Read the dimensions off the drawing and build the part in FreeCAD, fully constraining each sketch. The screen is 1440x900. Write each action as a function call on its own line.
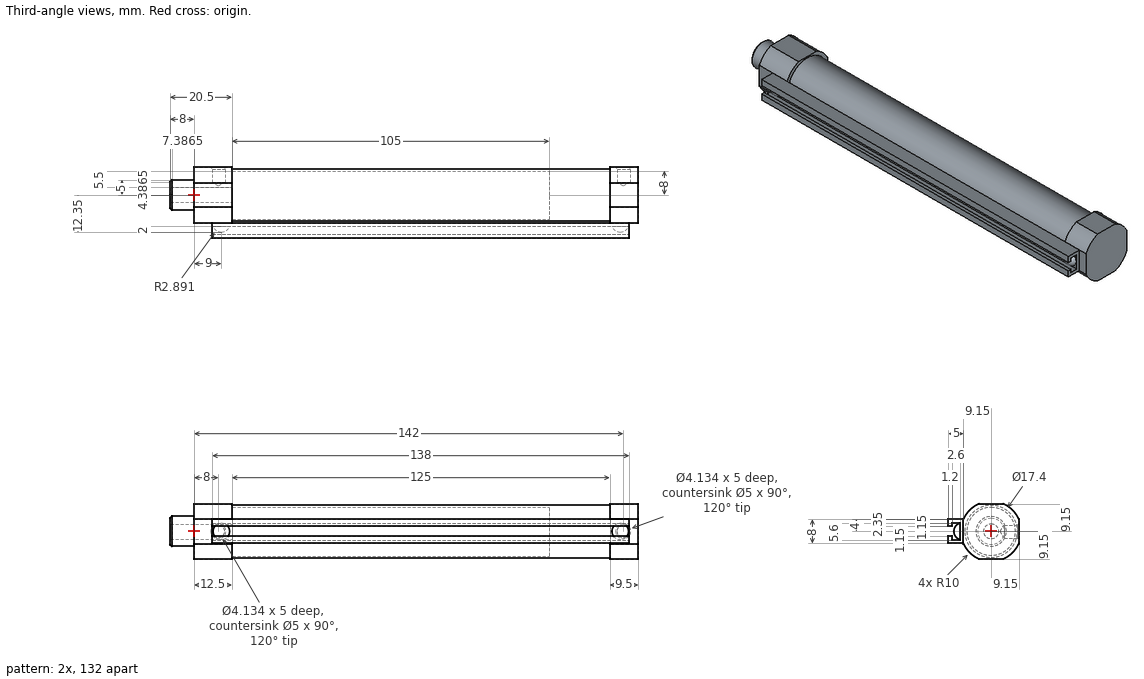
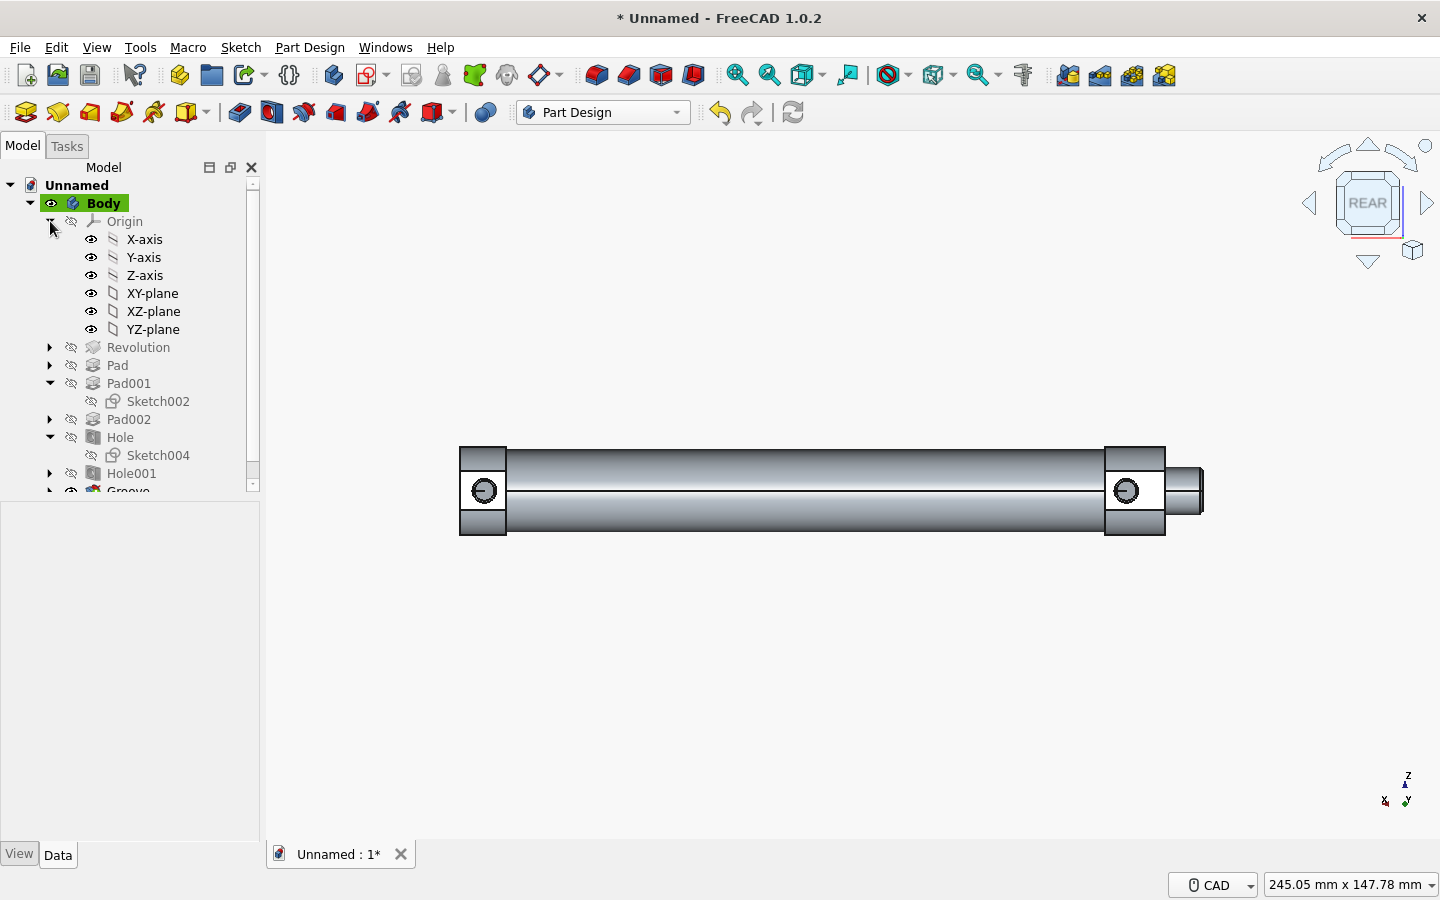
click(136, 329)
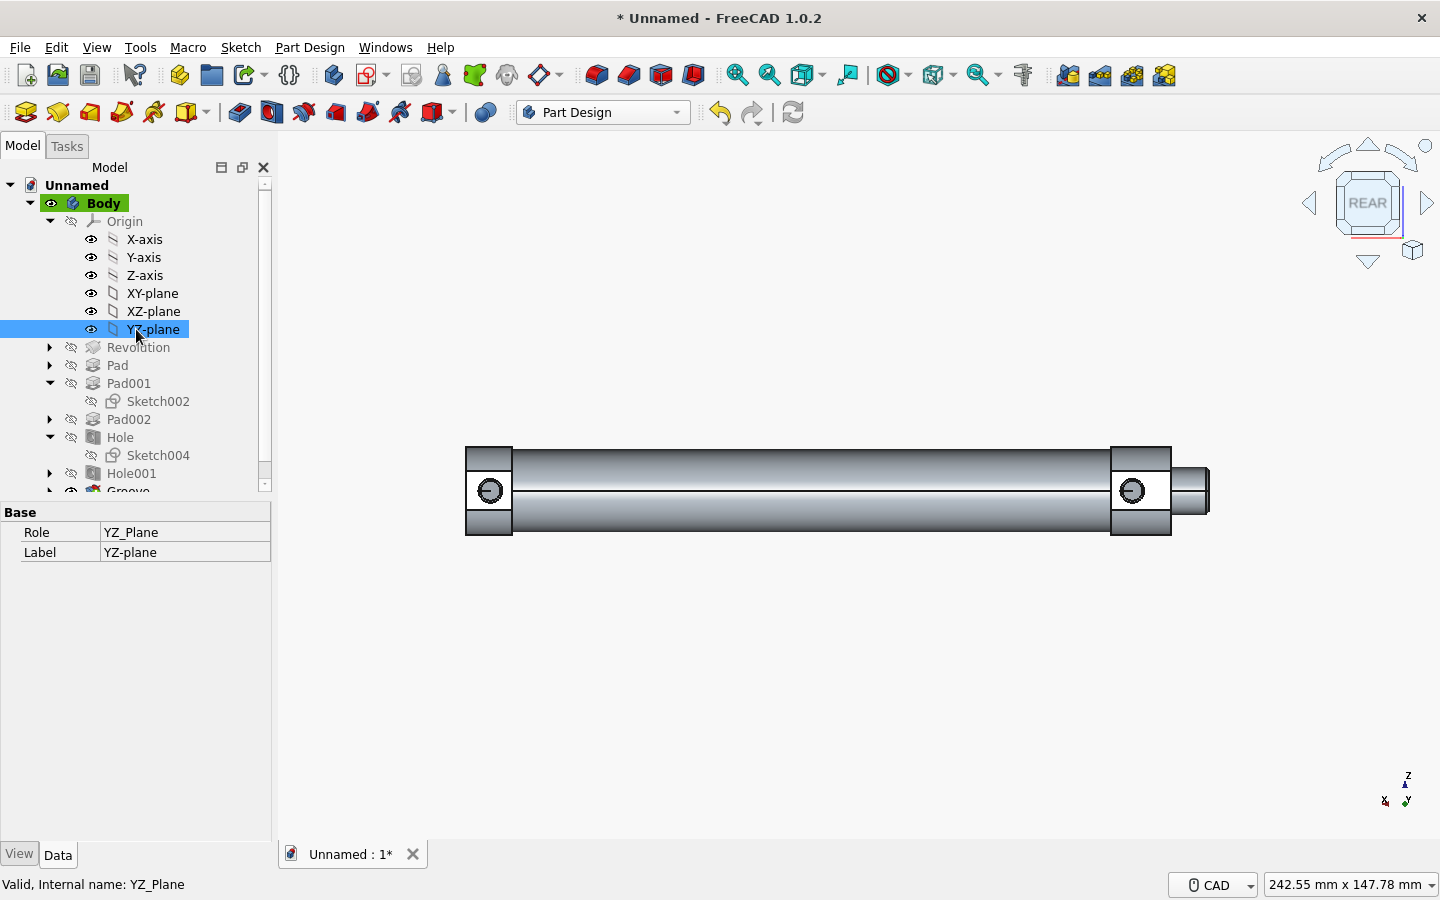
click(540, 76)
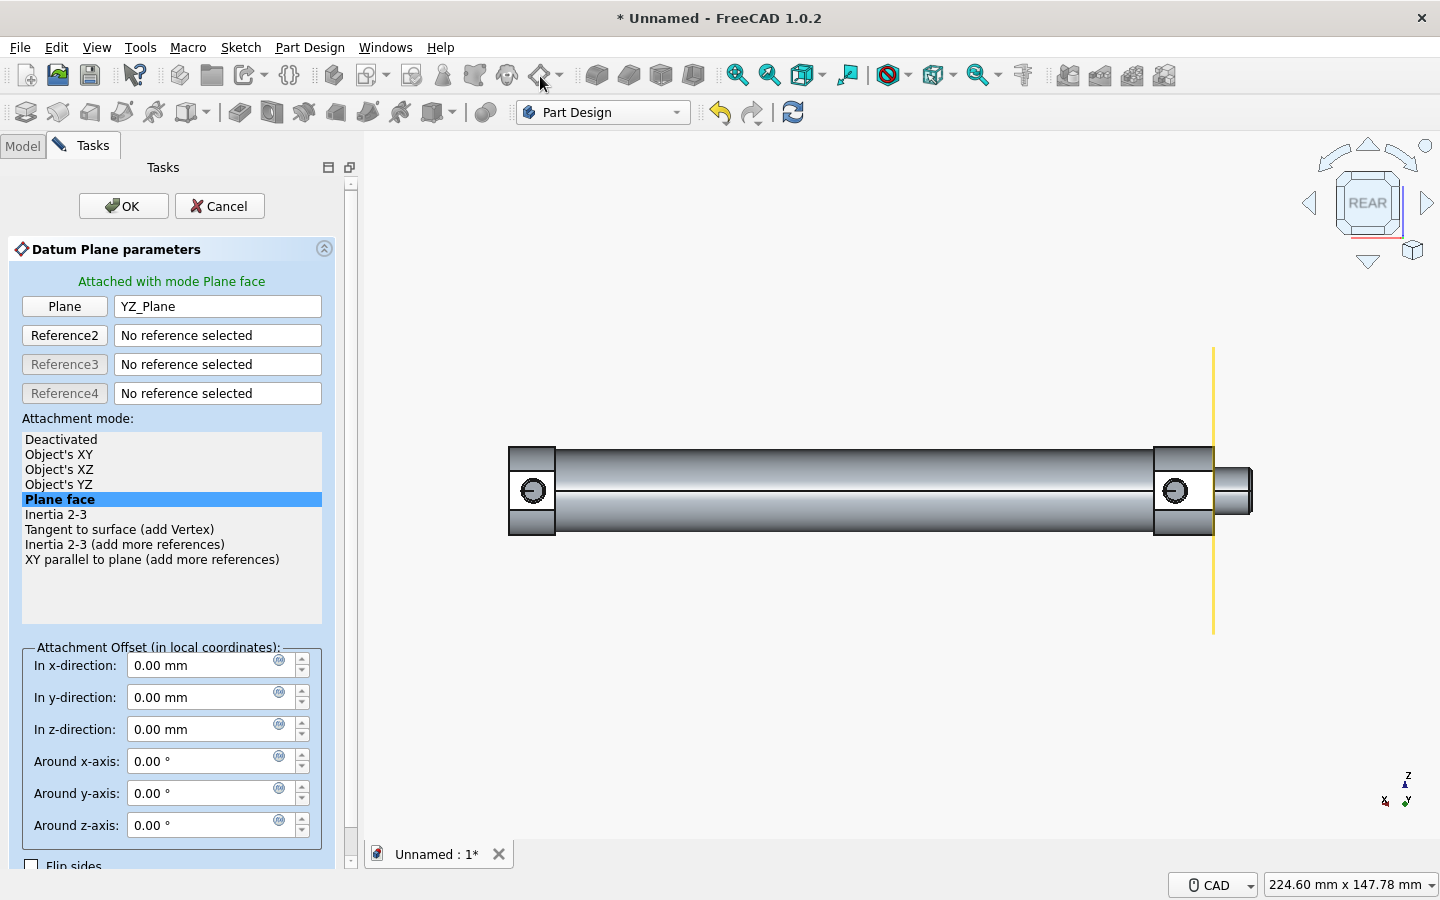
triple_click(210, 729)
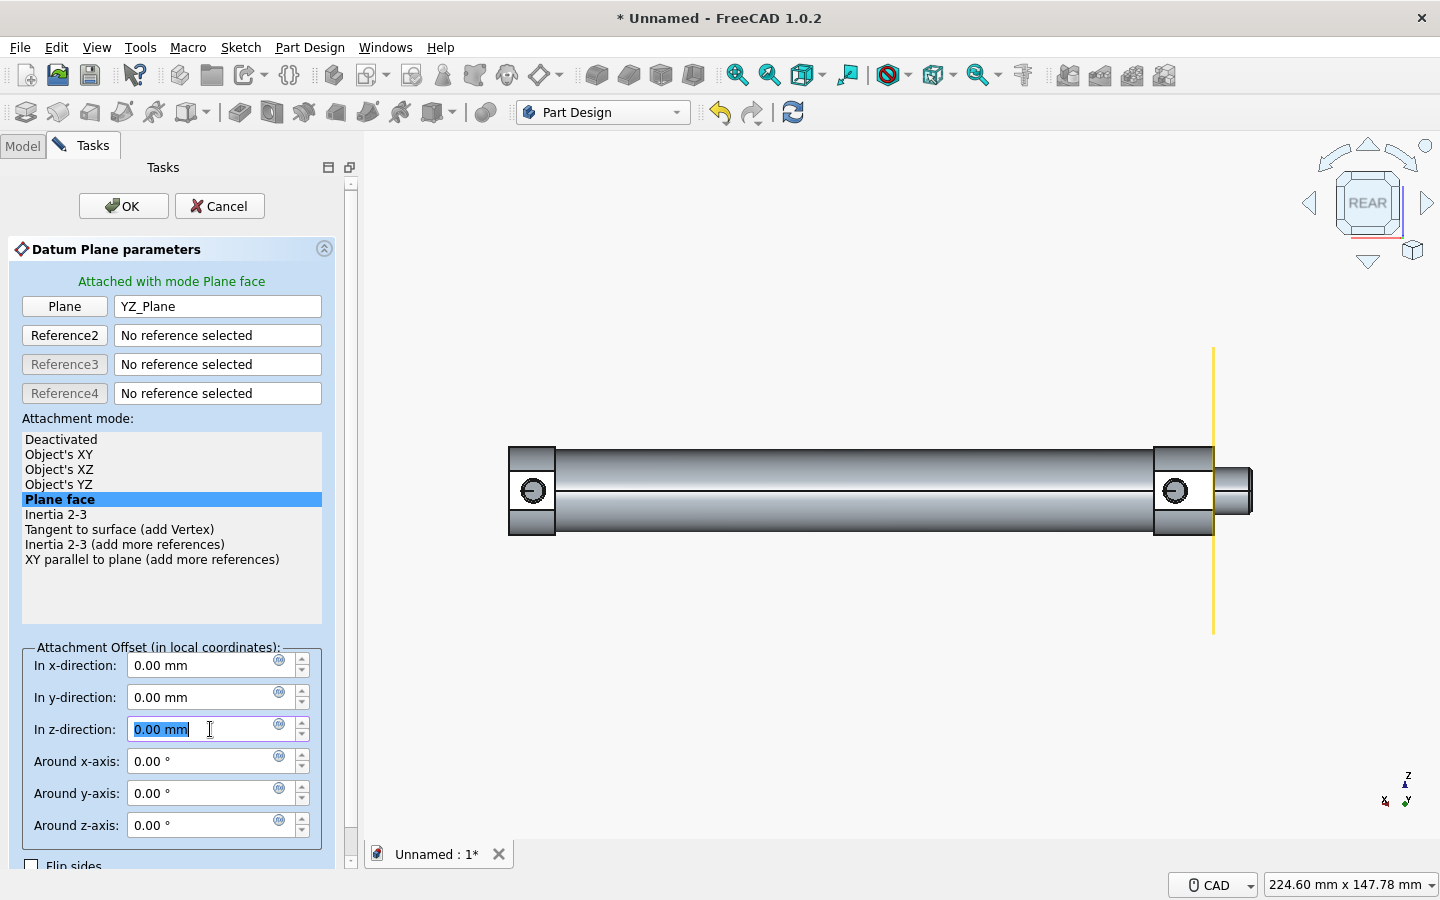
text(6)
key(Tab)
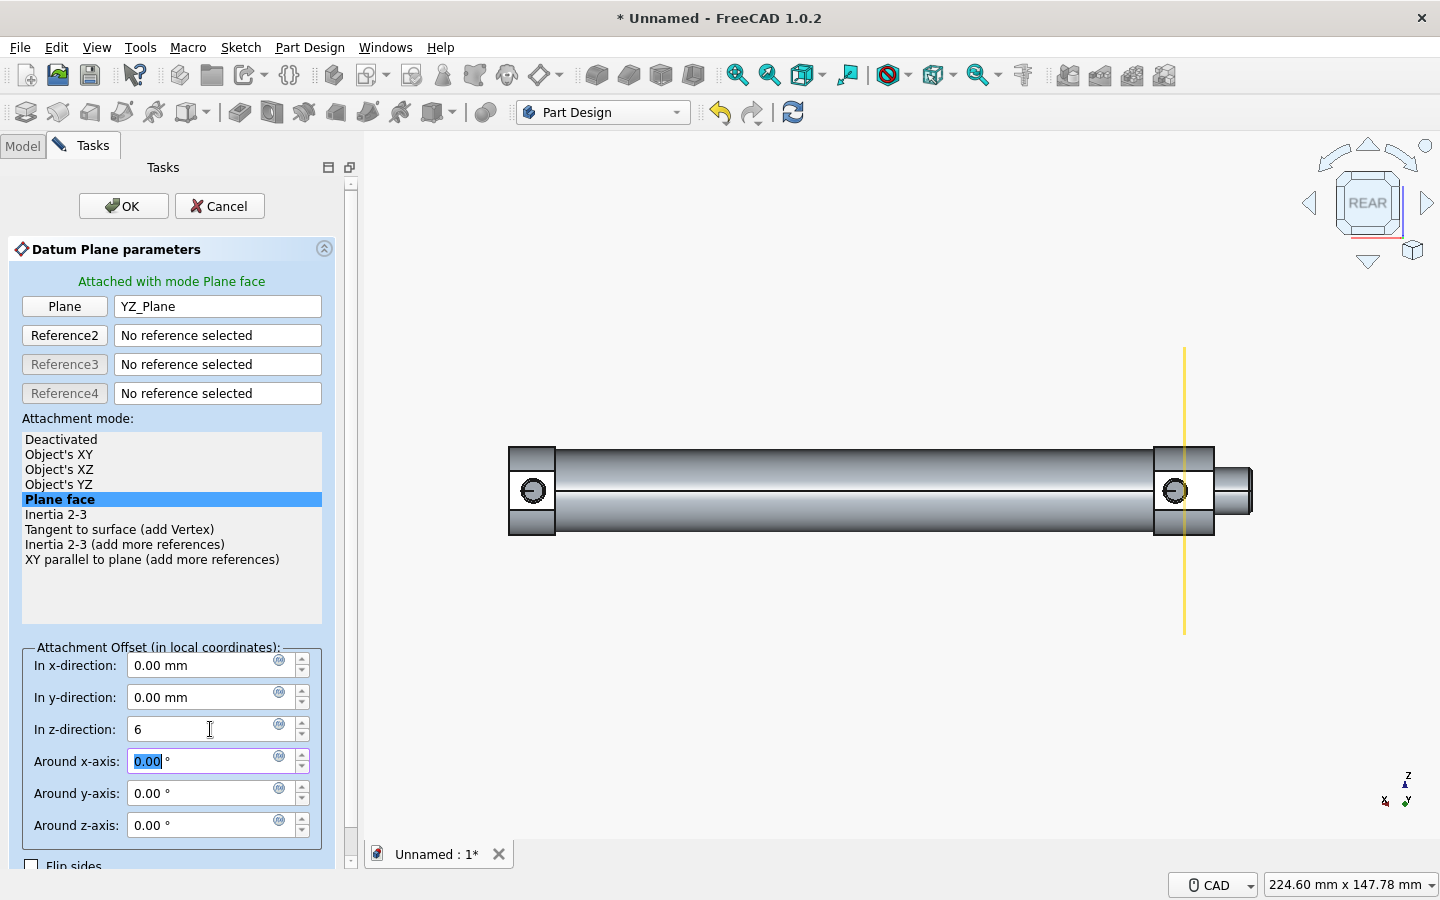
click(124, 206)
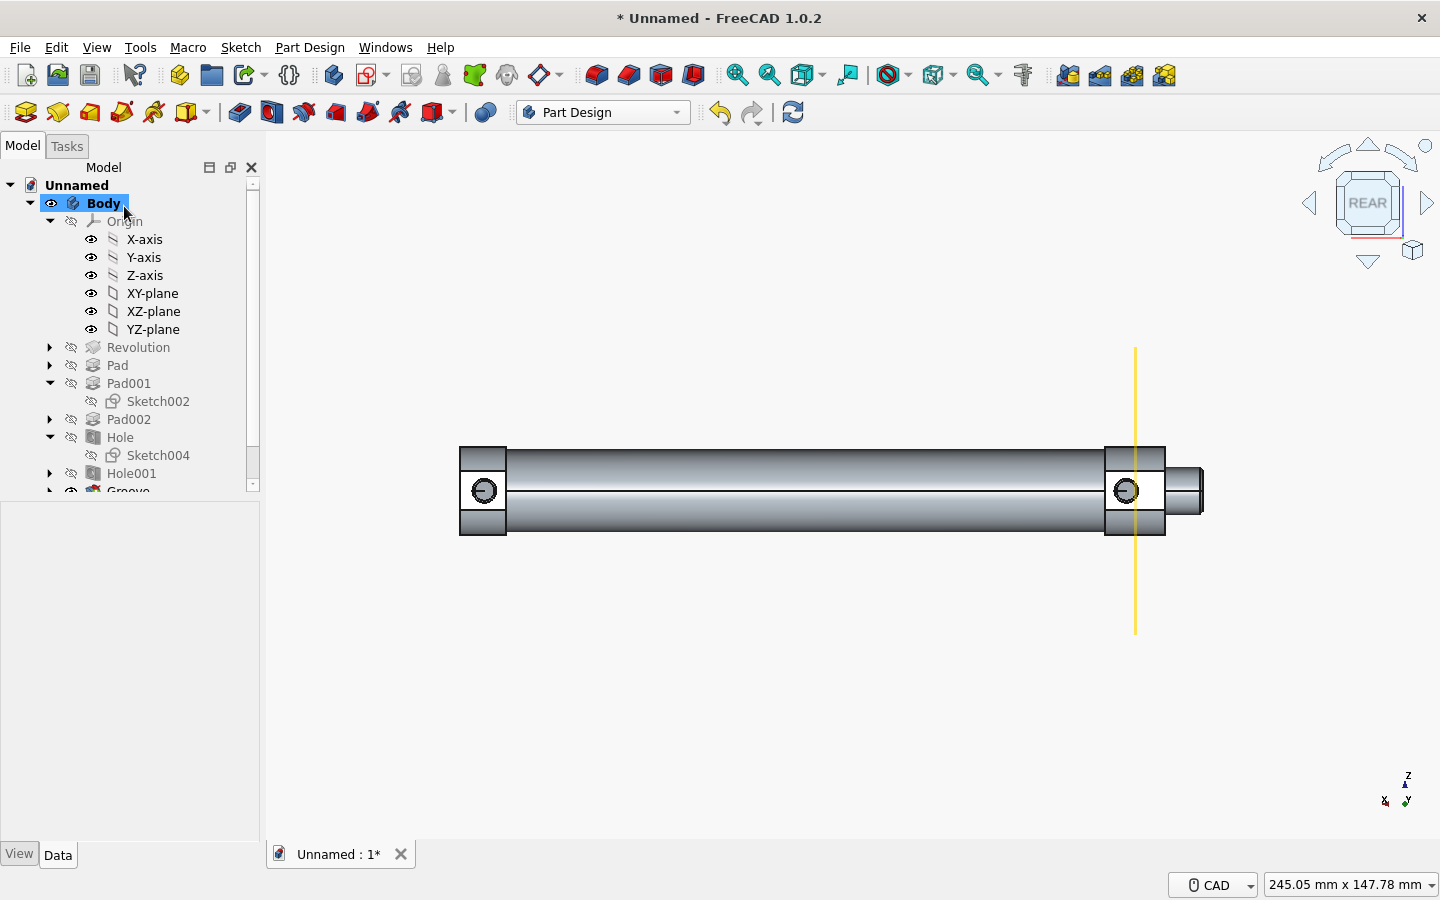
scroll(100, 343, down, 3)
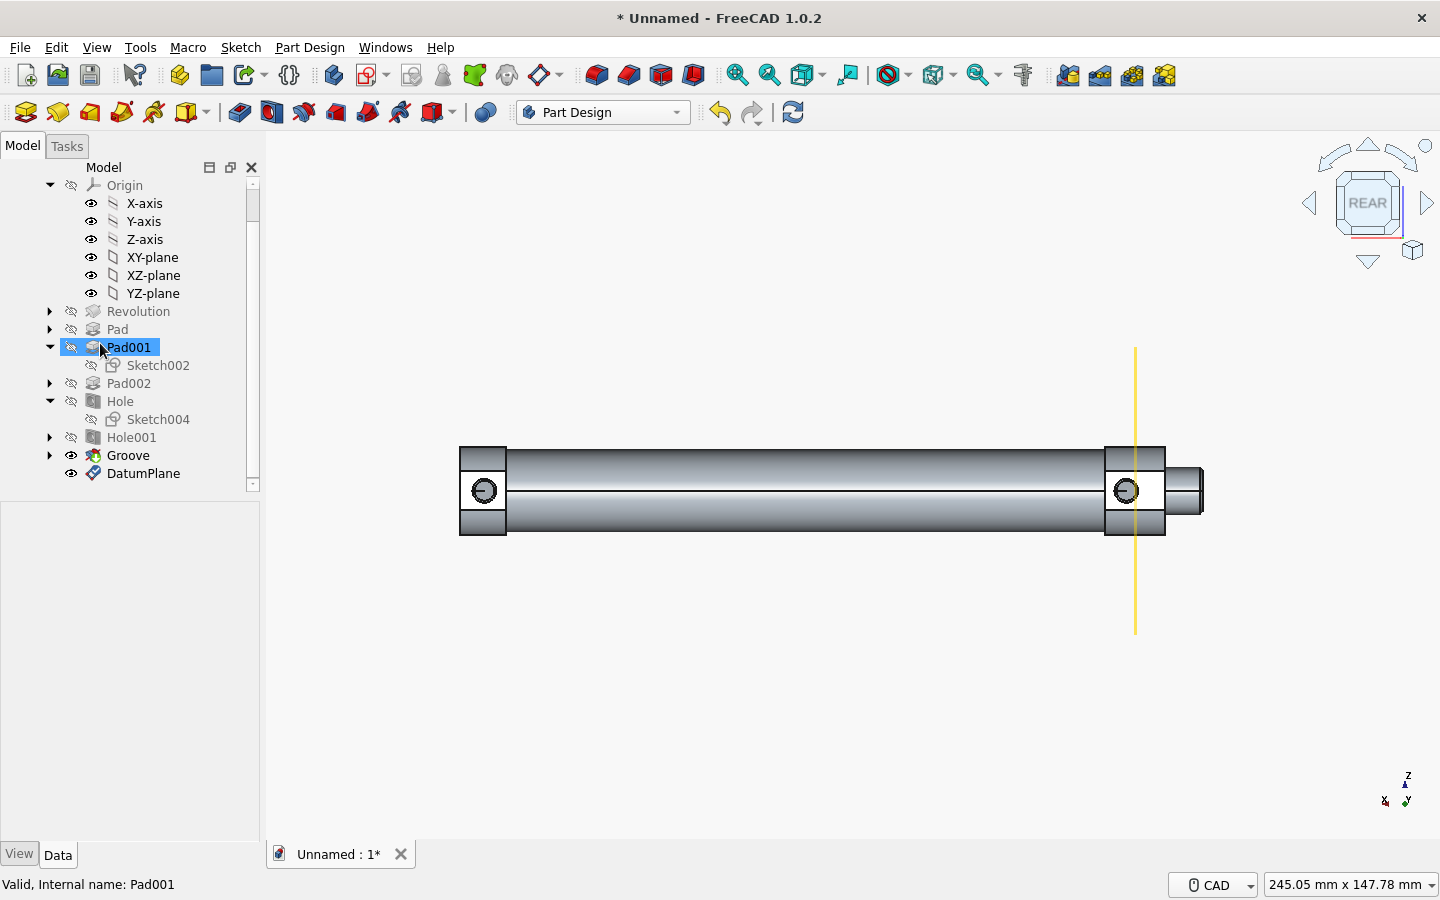
click(116, 473)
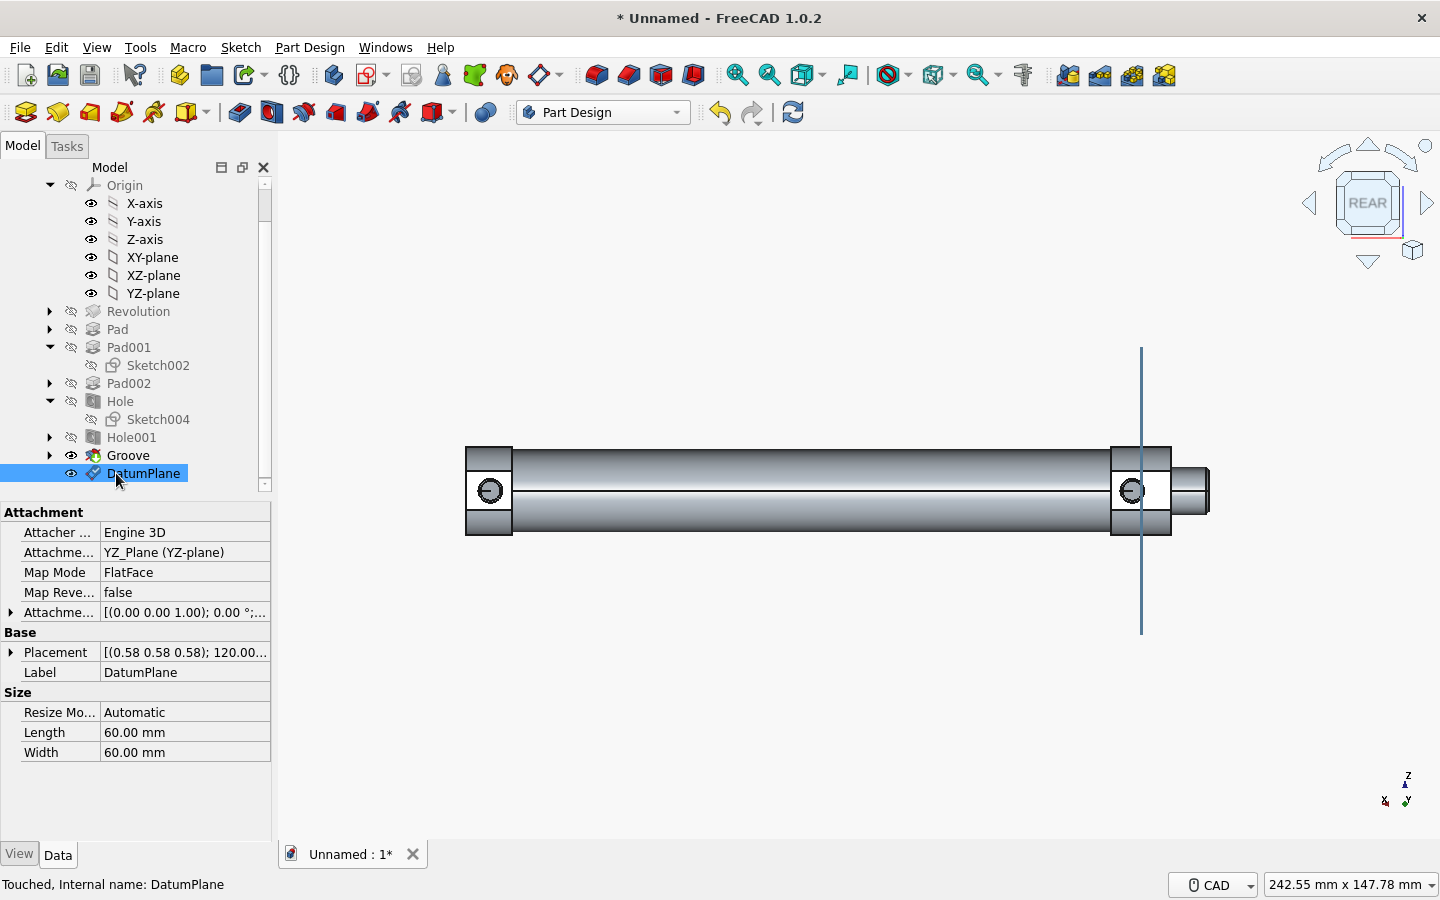
click(366, 76)